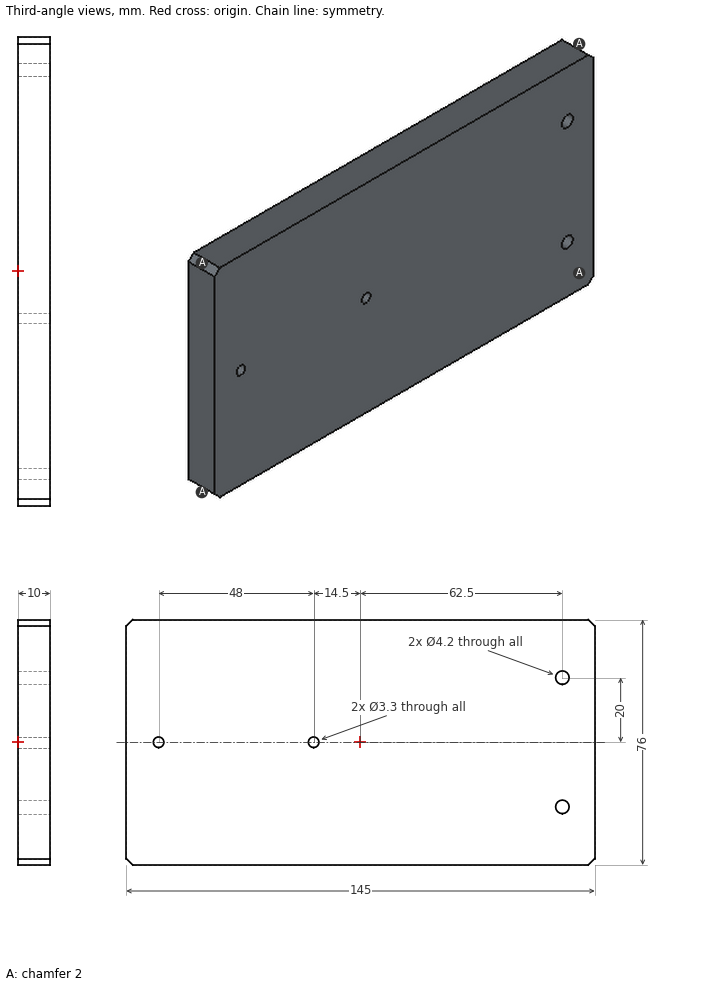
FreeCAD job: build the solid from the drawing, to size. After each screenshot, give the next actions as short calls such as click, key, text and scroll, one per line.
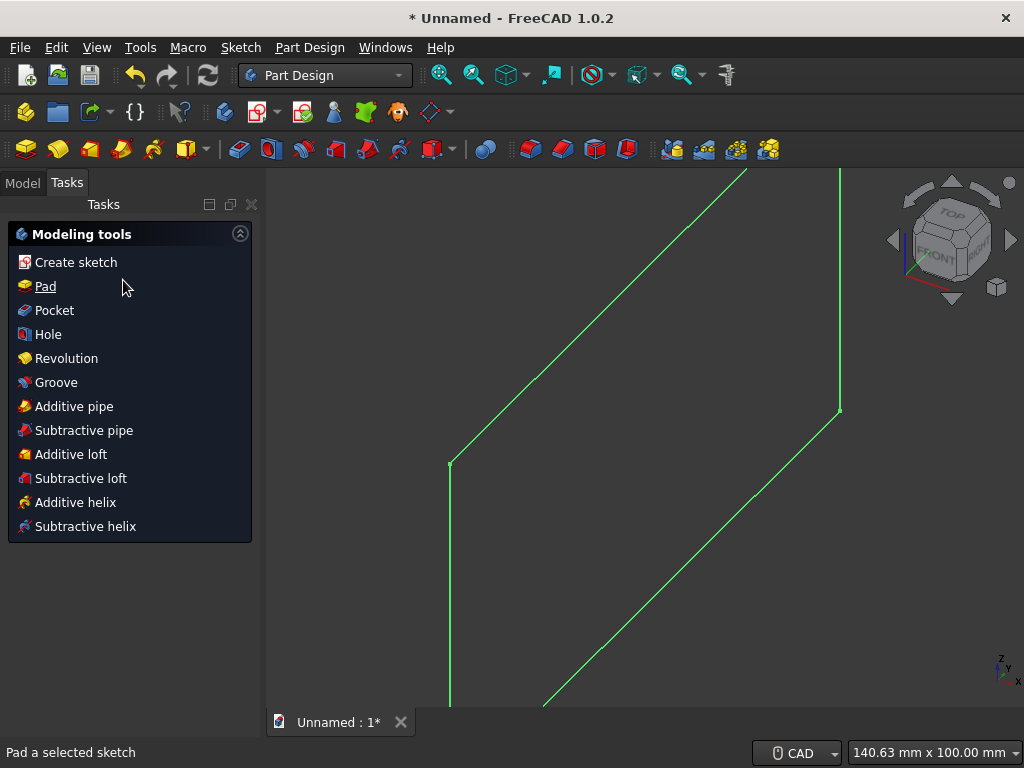
click(26, 150)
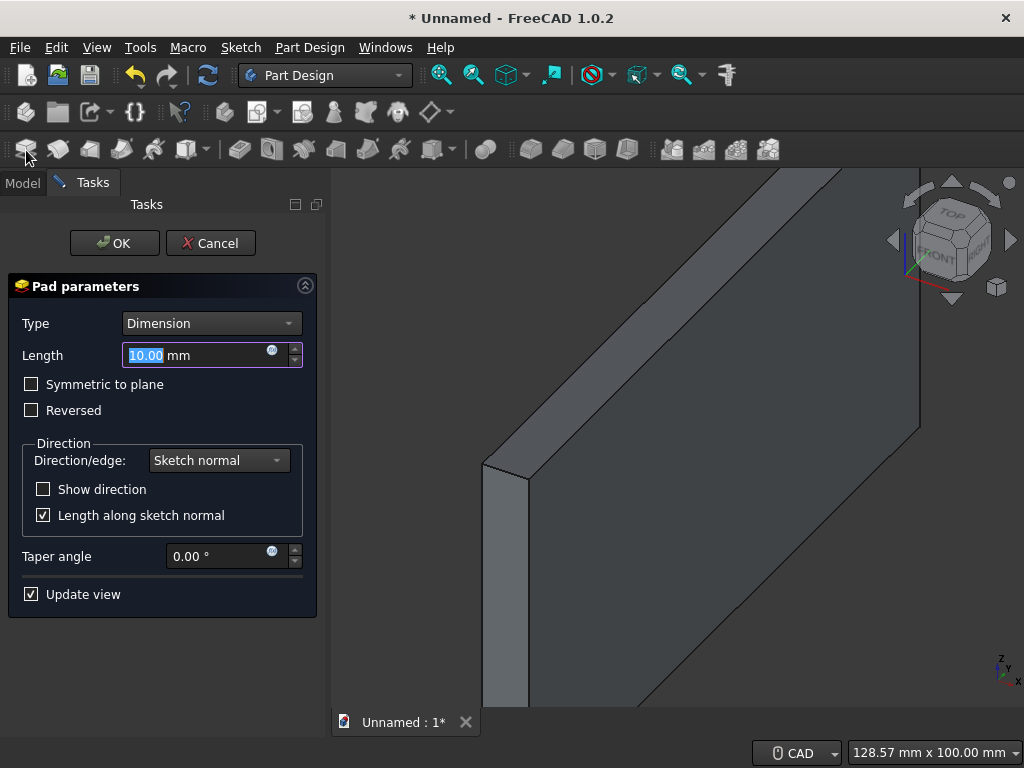
text(10)
key(Tab)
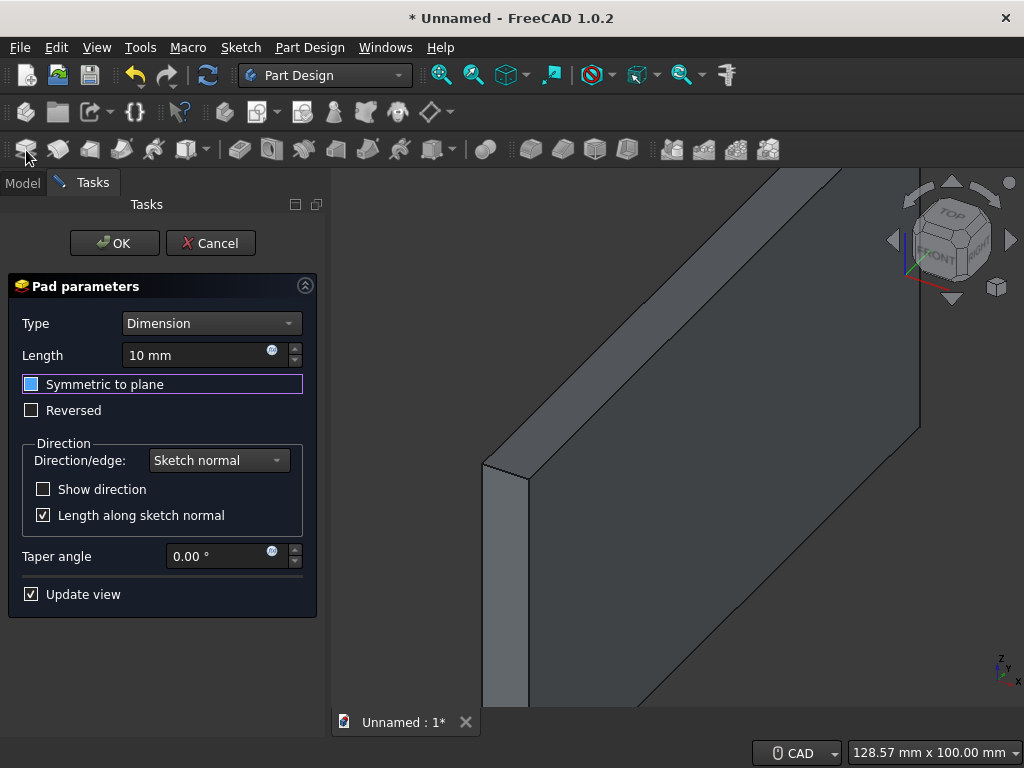
click(115, 243)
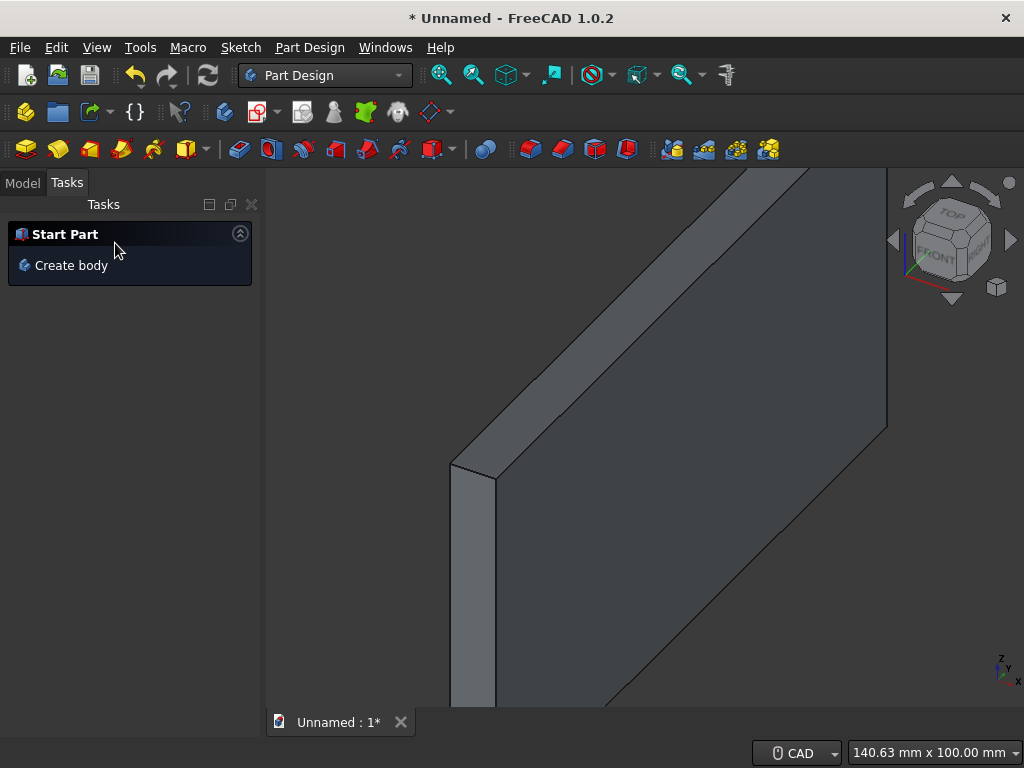
key(v)
key(f)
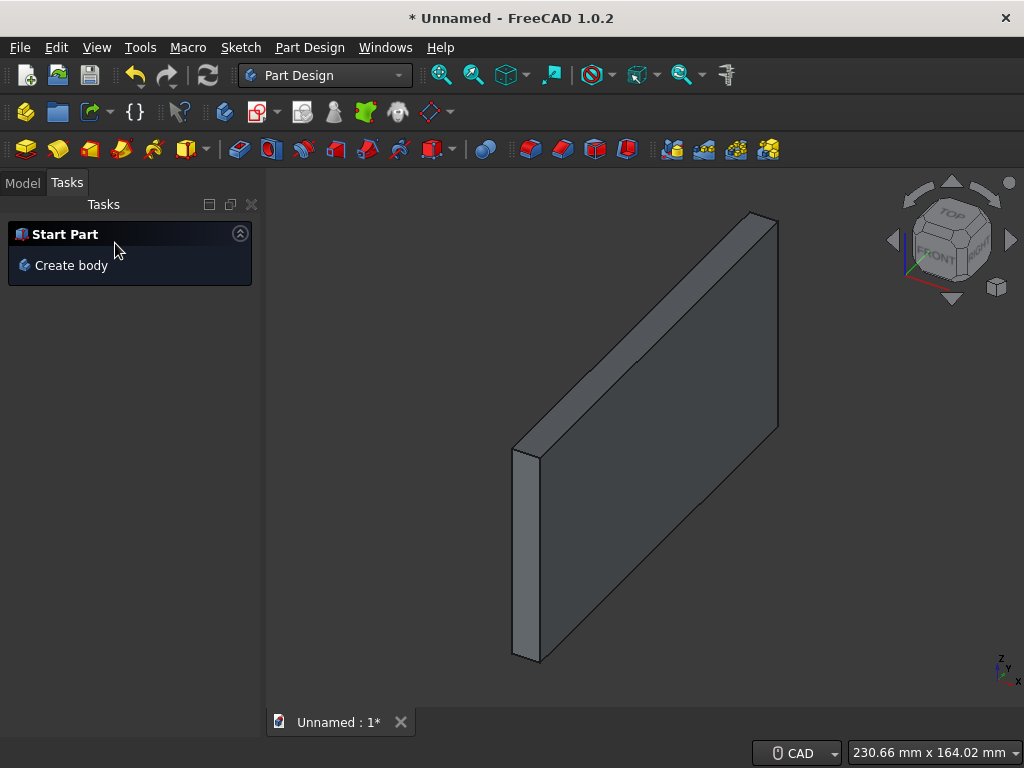
key(6)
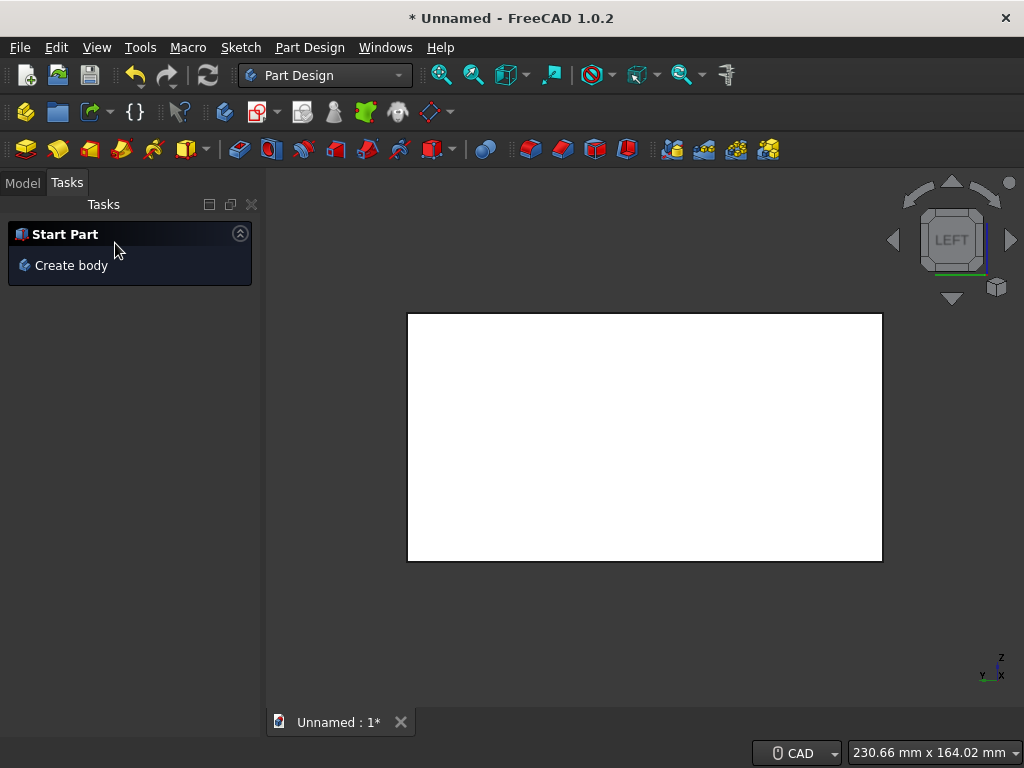
click(577, 436)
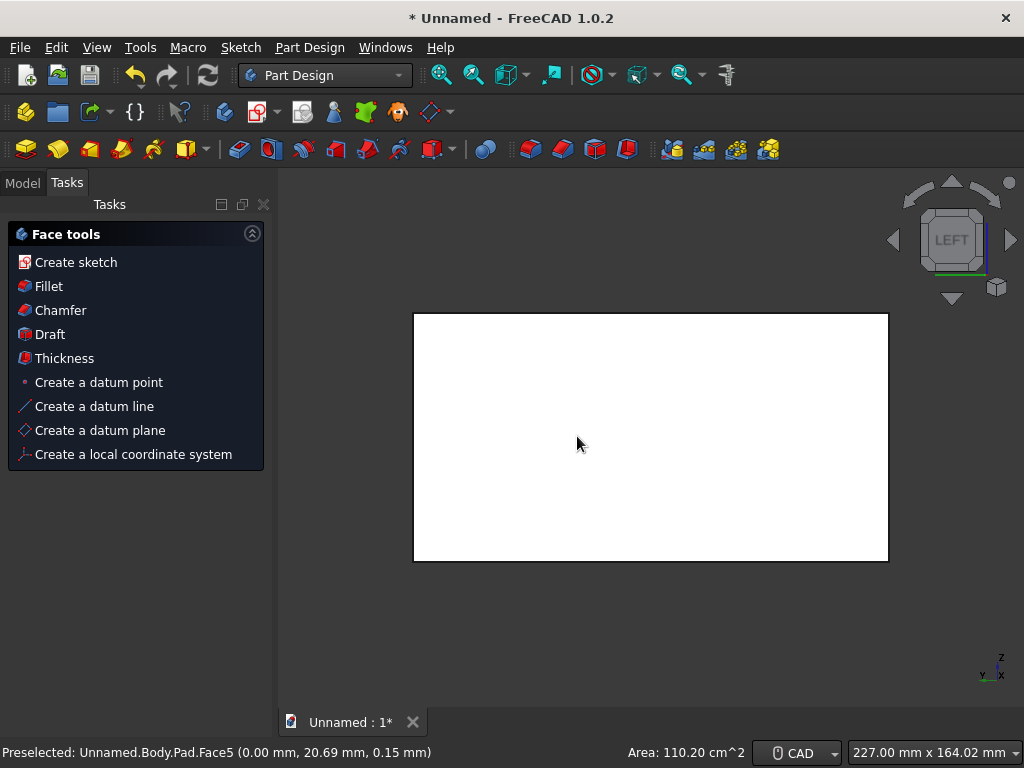
click(258, 112)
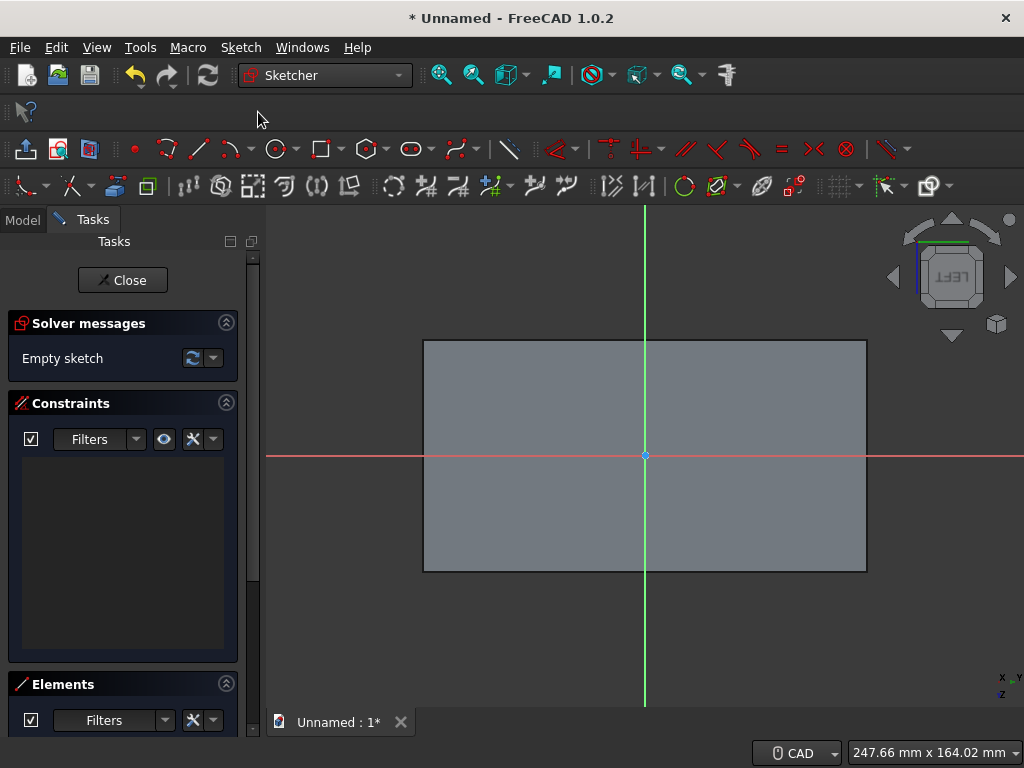
scroll(859, 456, up, 4)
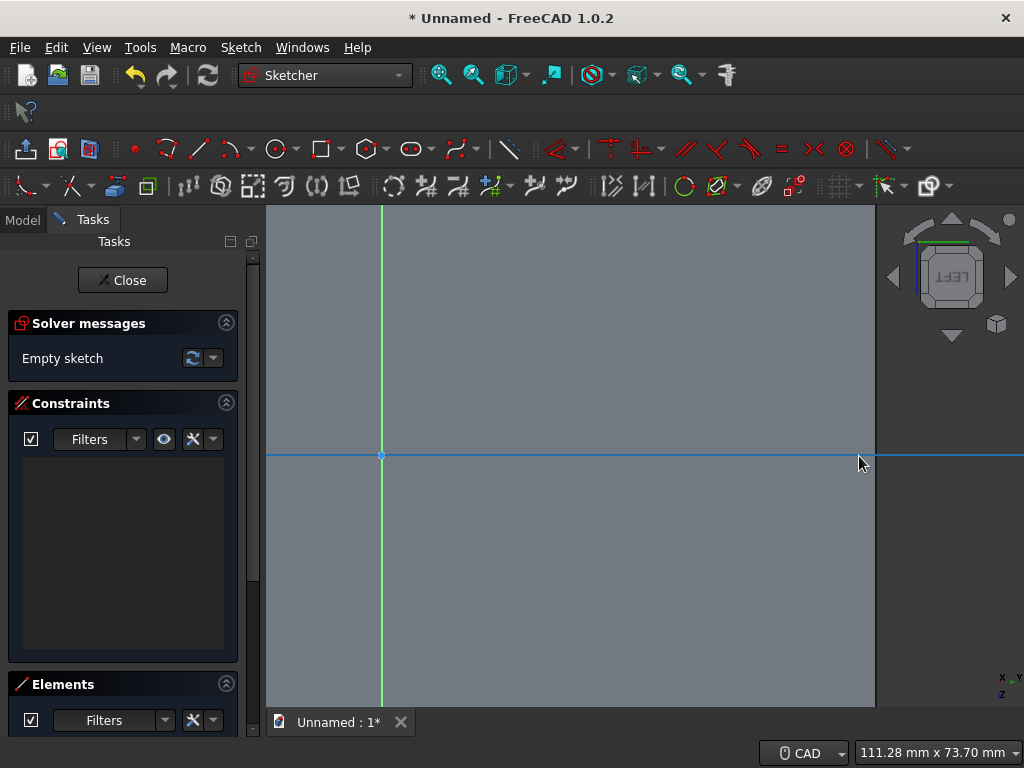
key(g)
key(c)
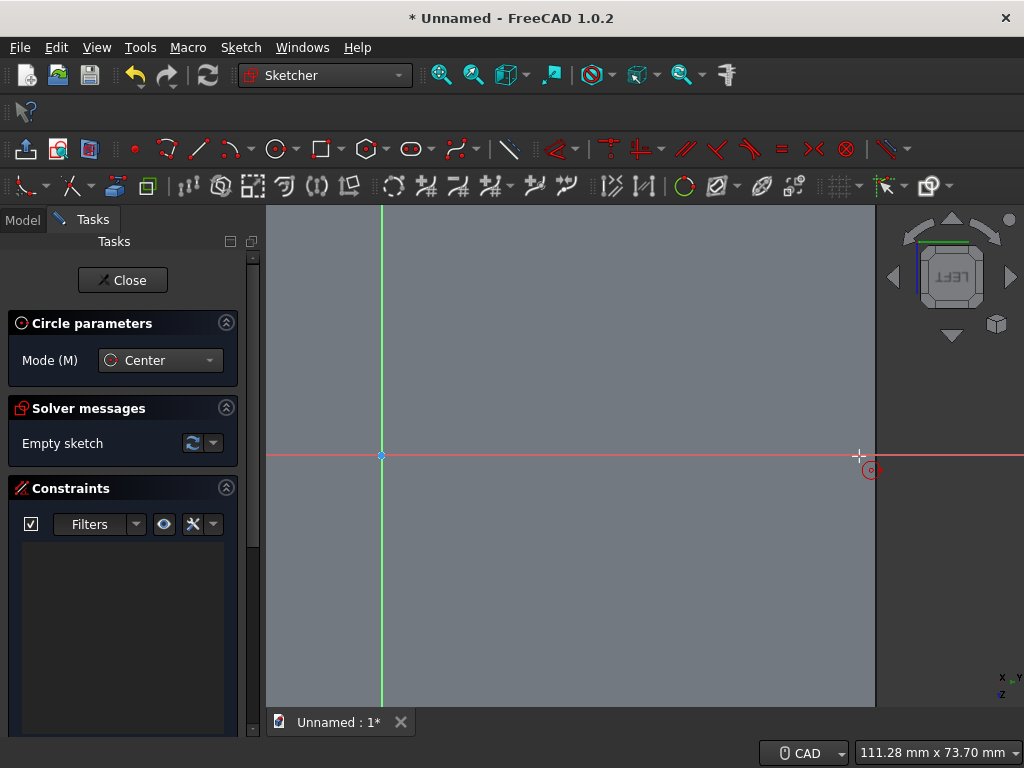
scroll(808, 592, up, 3)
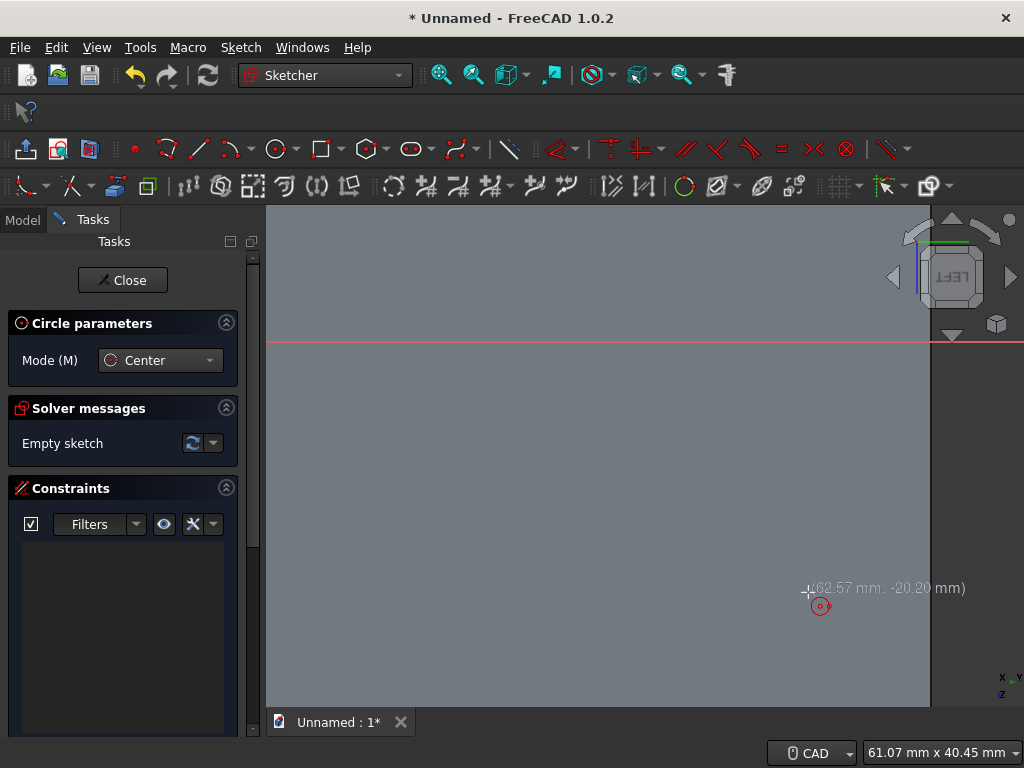
click(807, 591)
click(825, 572)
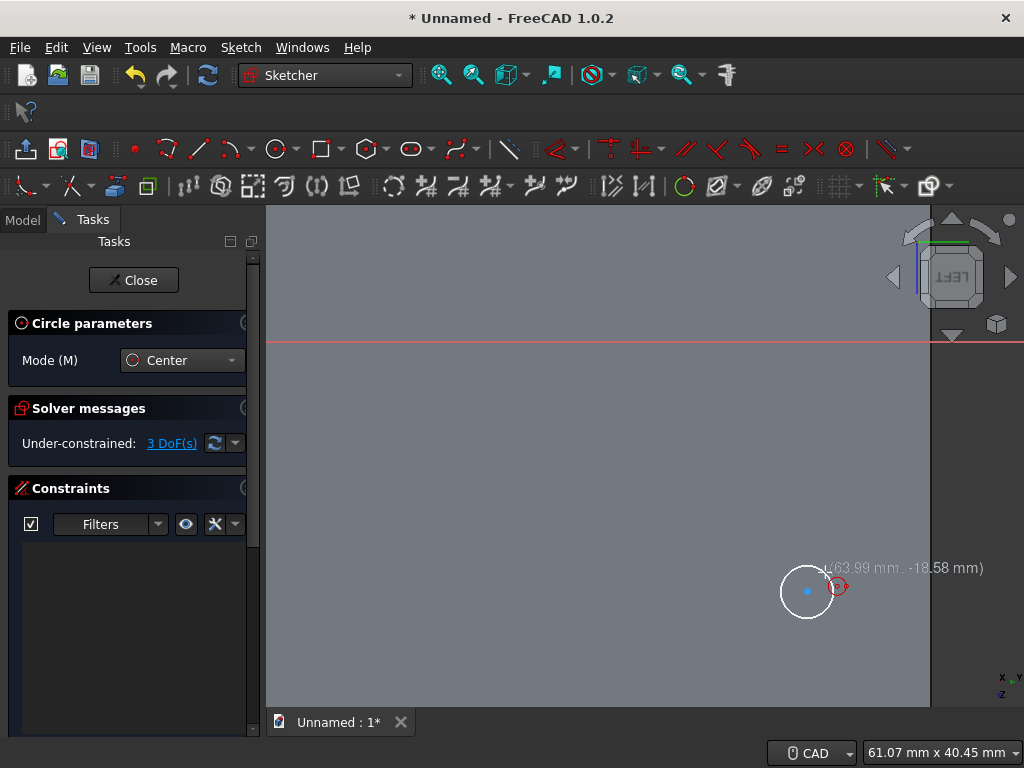
scroll(753, 594, down, 3)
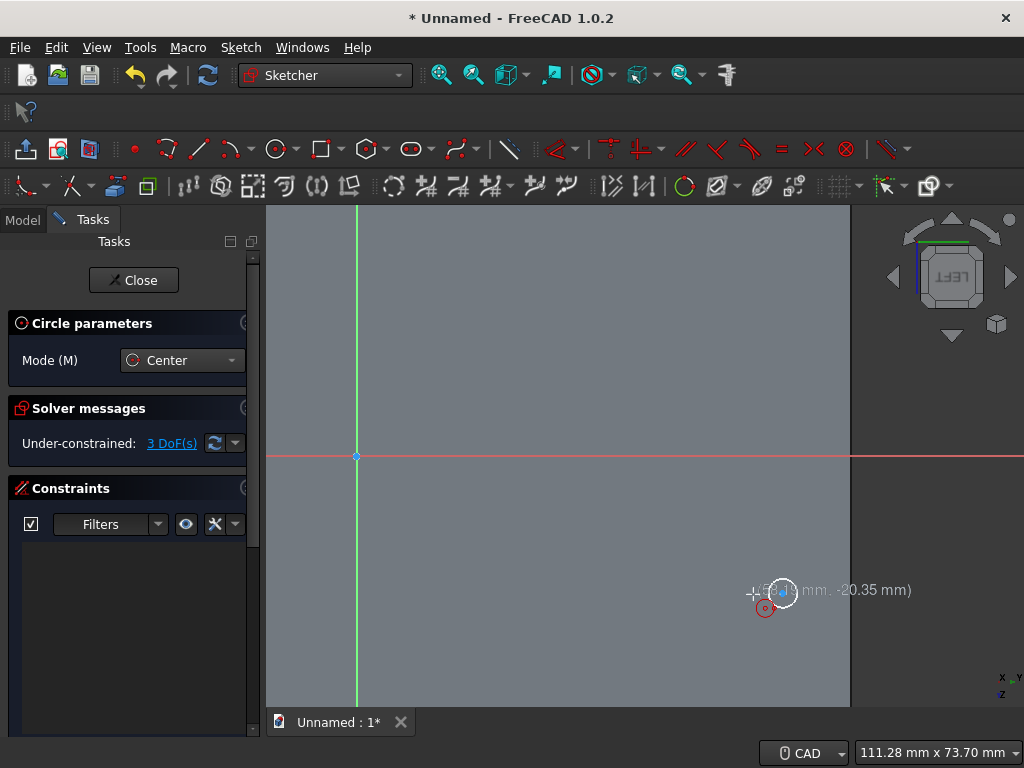
scroll(783, 320, up, 3)